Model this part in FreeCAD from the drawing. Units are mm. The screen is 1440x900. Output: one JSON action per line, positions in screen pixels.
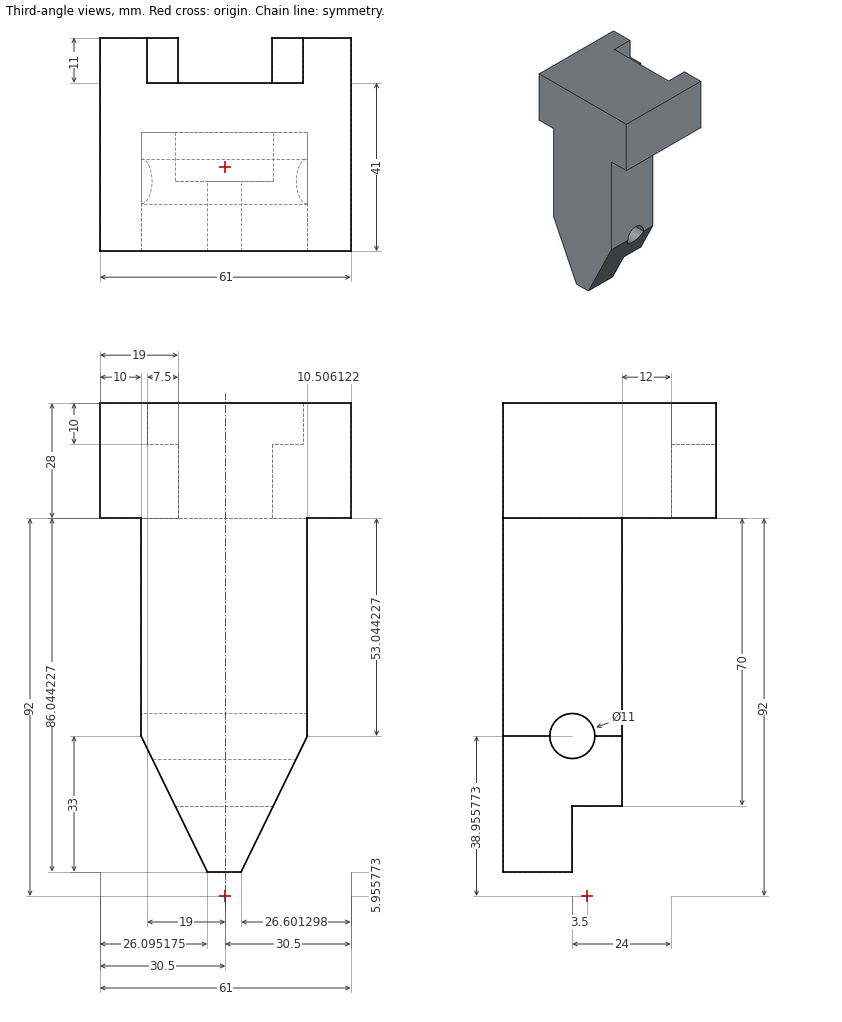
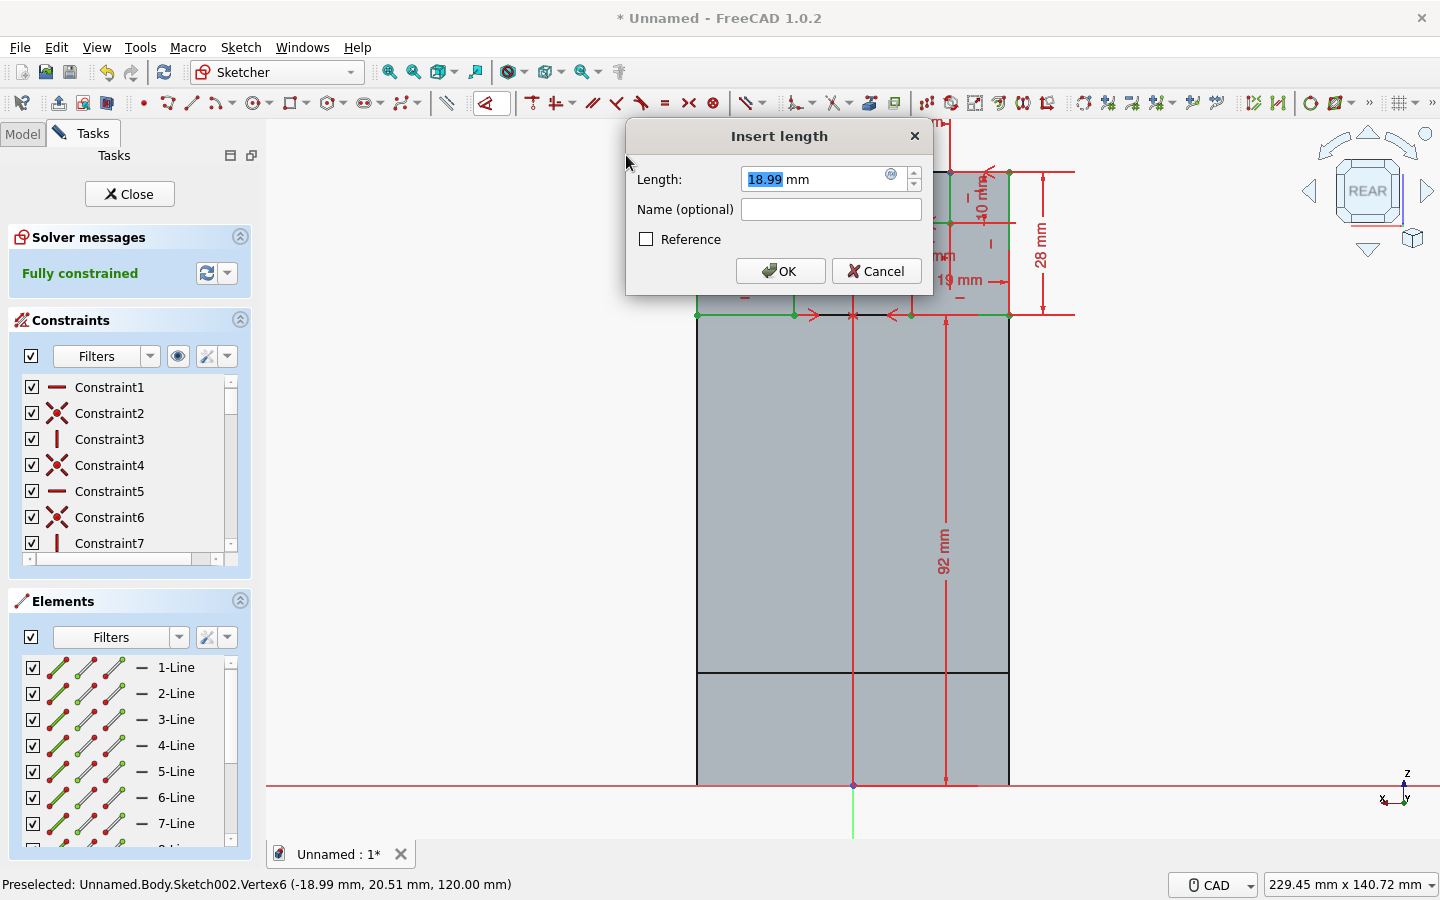
{"action": "type", "text": "19"}
{"action": "key", "text": "Return"}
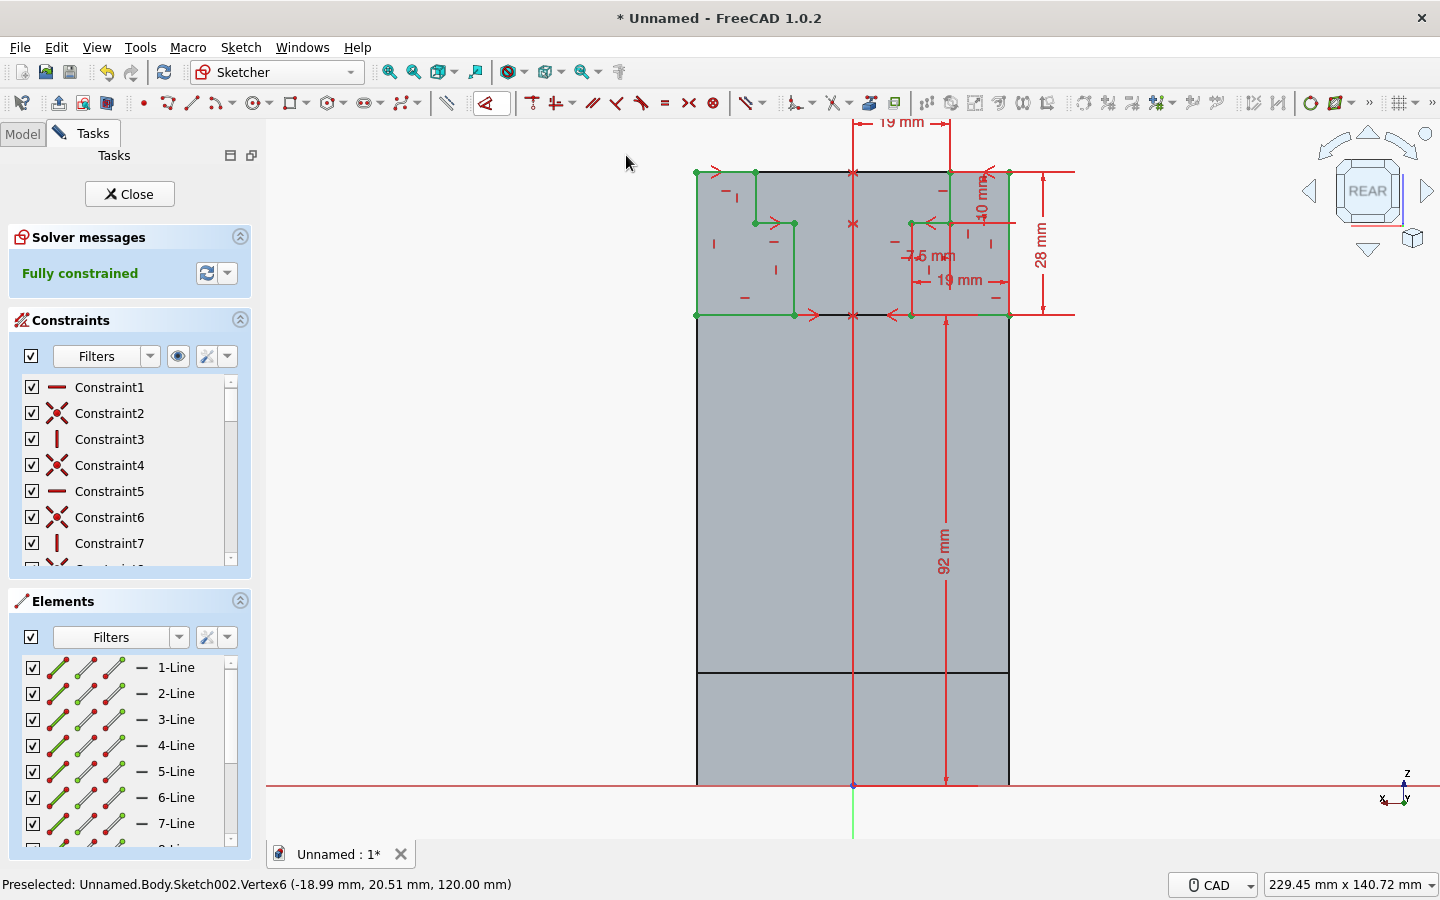
{"action": "left_click", "coordinate": [130, 194]}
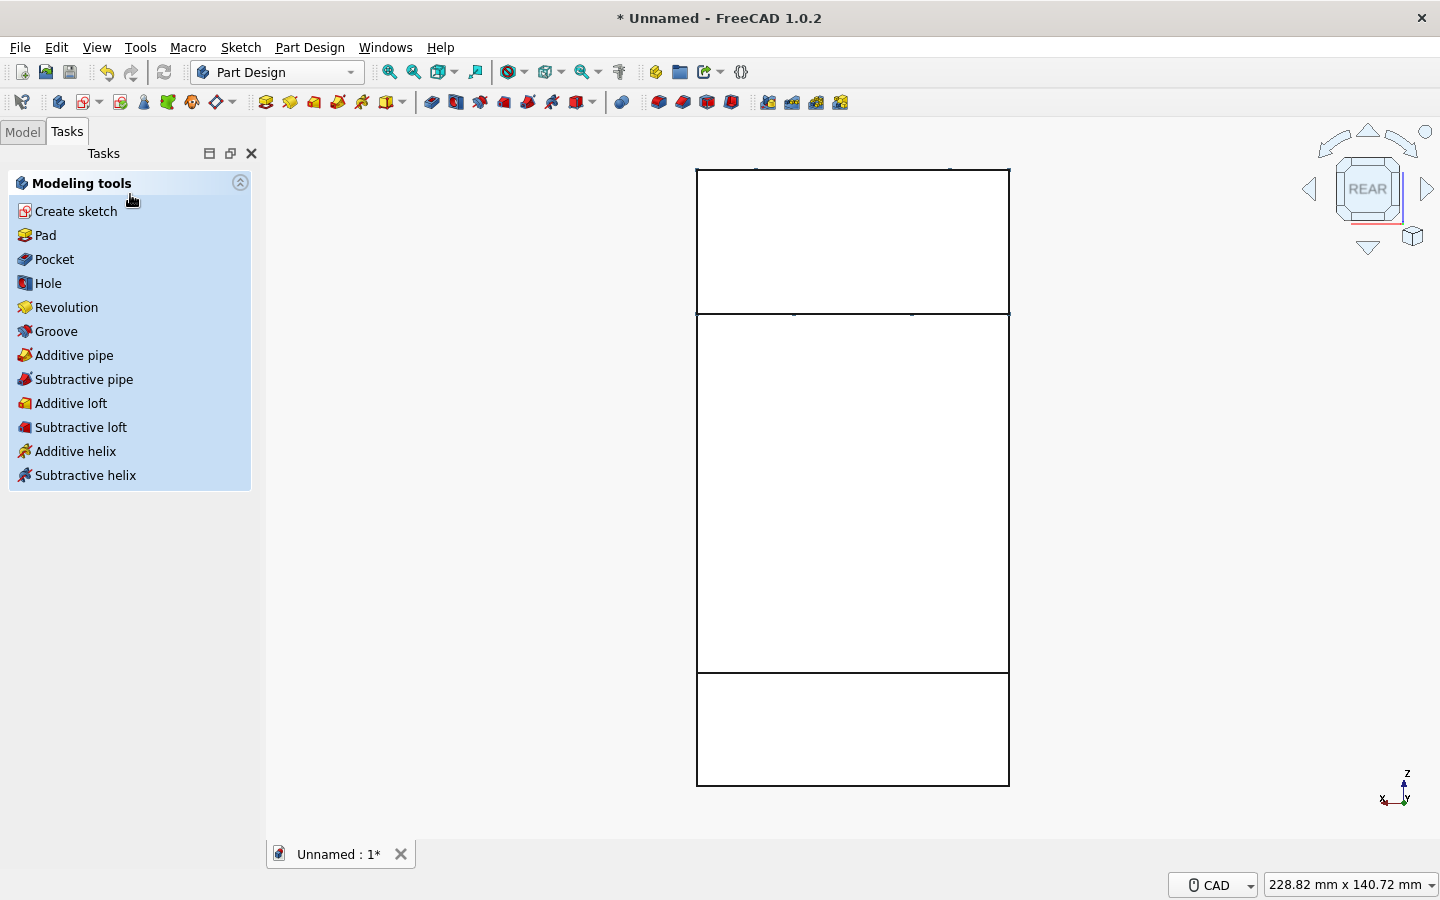
{"action": "left_click", "coordinate": [266, 102]}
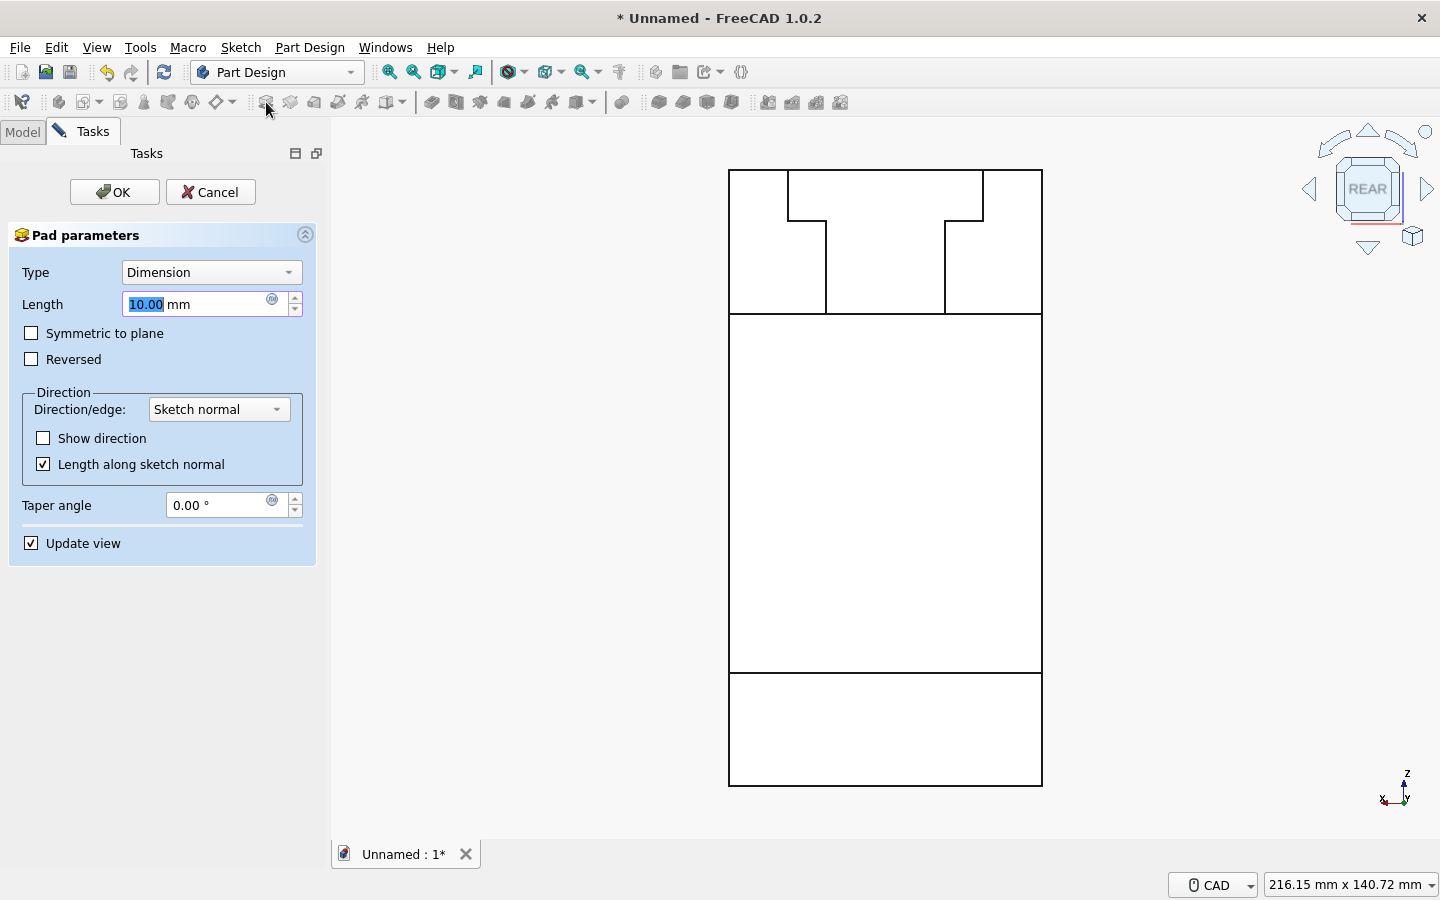
{"action": "type", "text": "11"}
{"action": "key", "text": "Tab"}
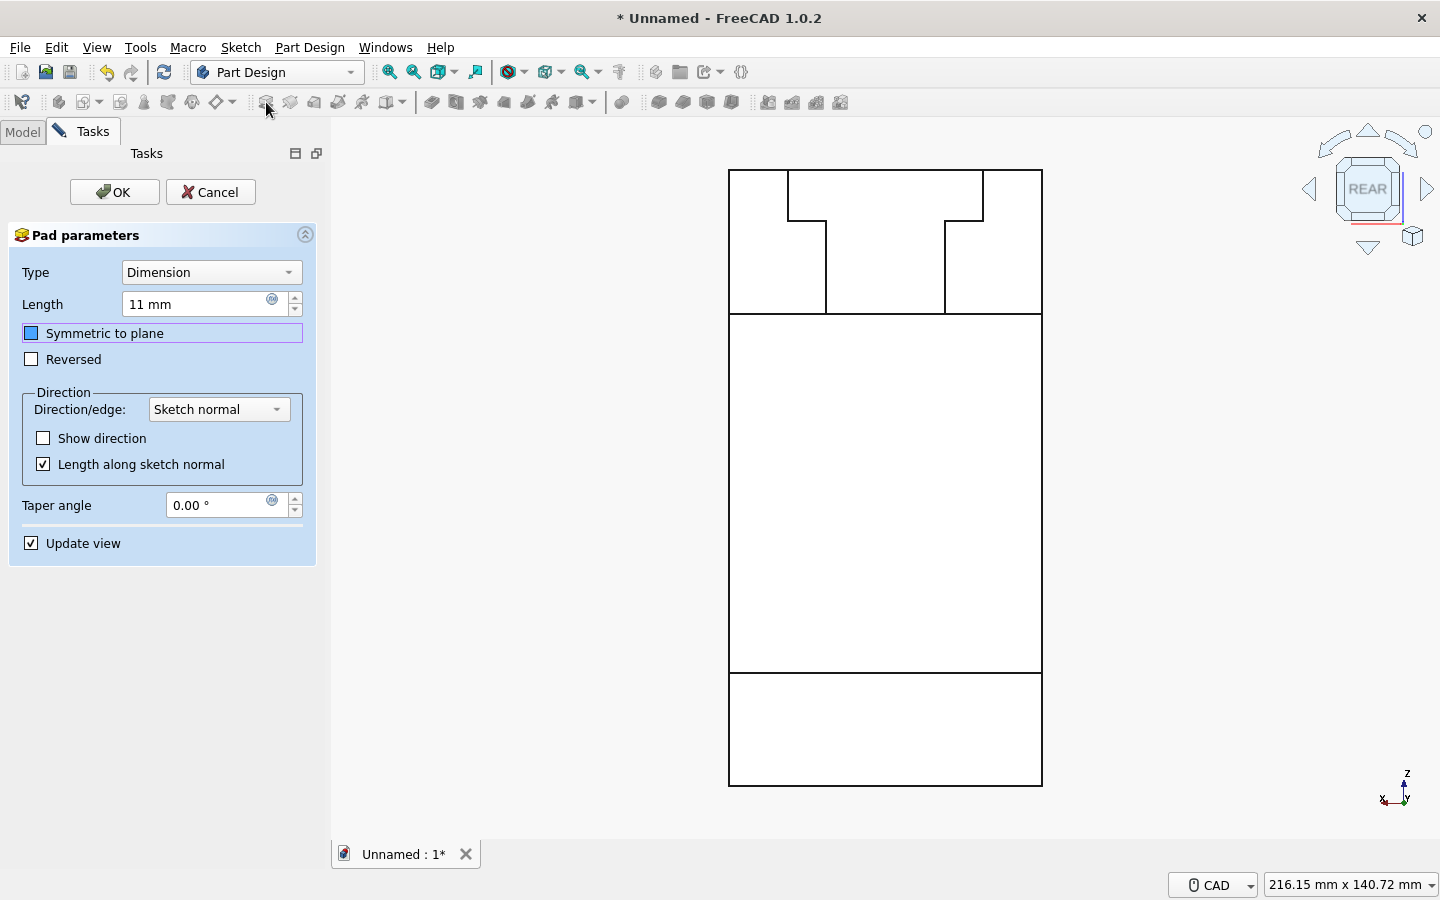
{"action": "left_click", "coordinate": [115, 192]}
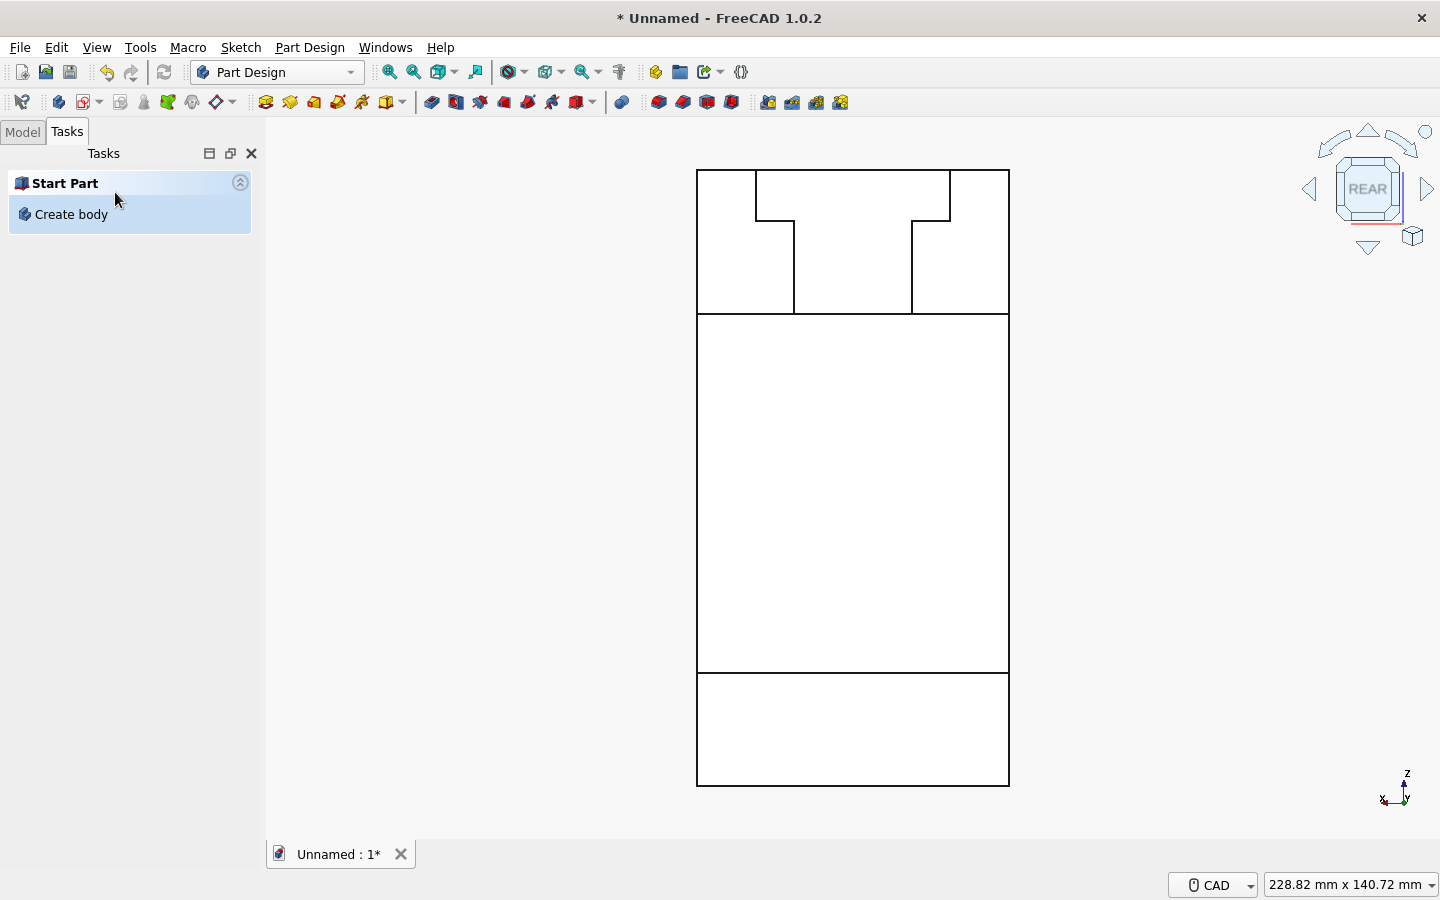
{"action": "left_click", "coordinate": [84, 102]}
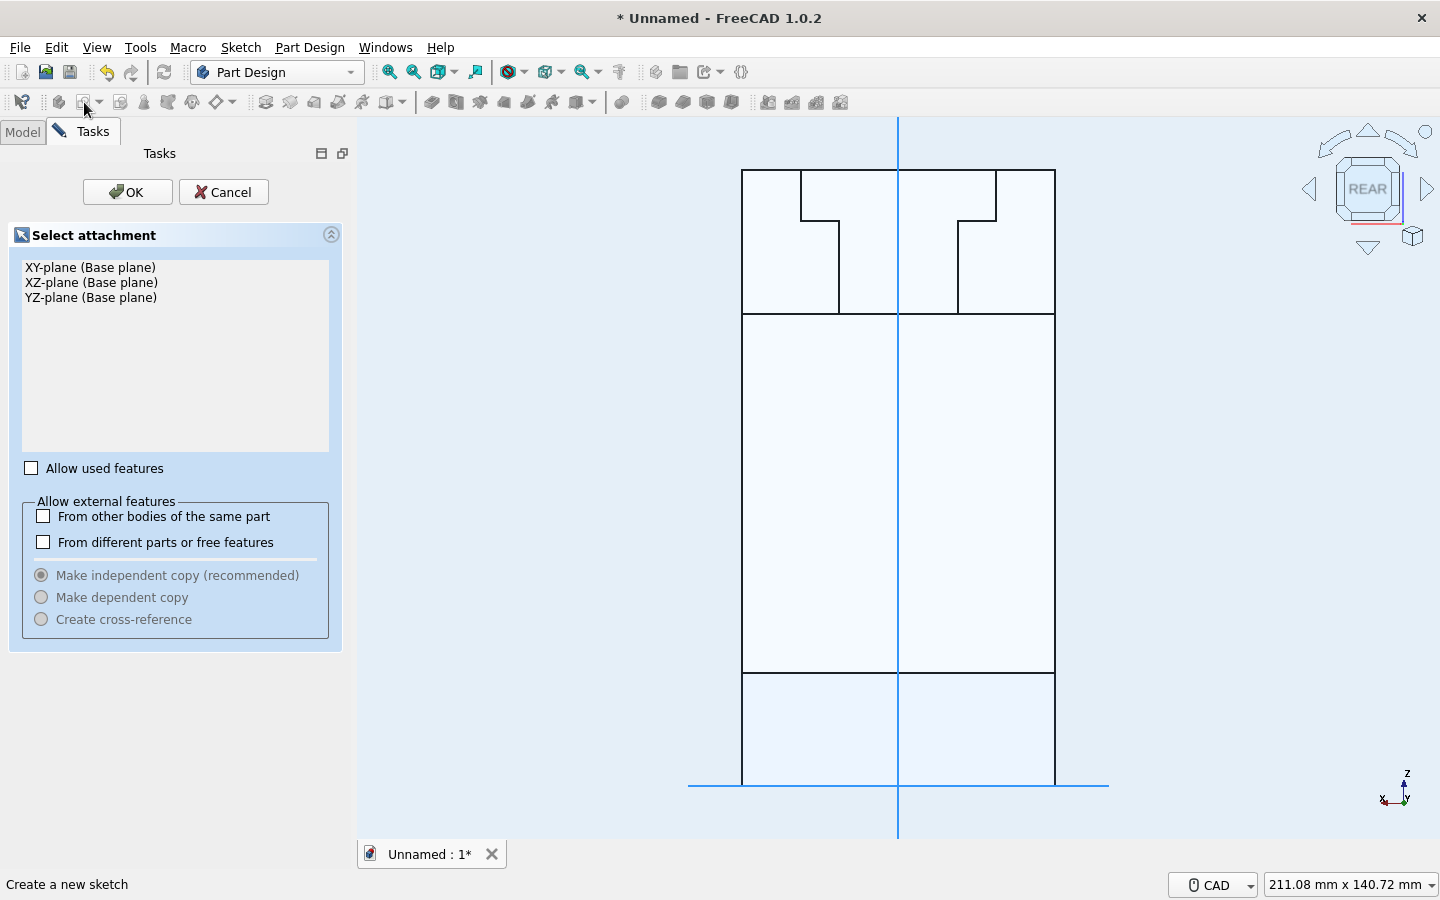
{"action": "left_click", "coordinate": [82, 282]}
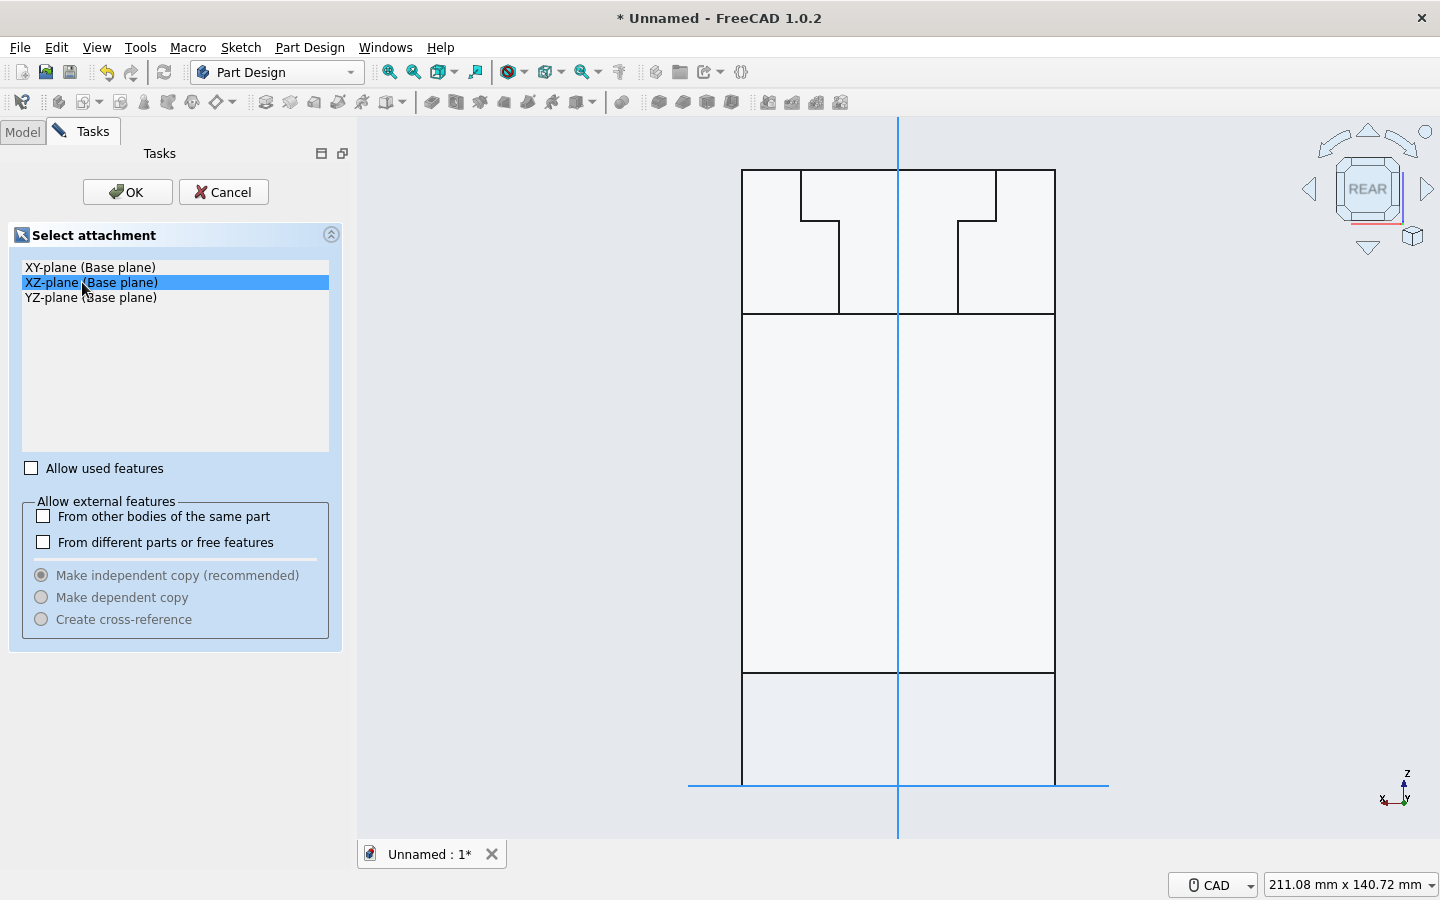
{"action": "left_click", "coordinate": [128, 192]}